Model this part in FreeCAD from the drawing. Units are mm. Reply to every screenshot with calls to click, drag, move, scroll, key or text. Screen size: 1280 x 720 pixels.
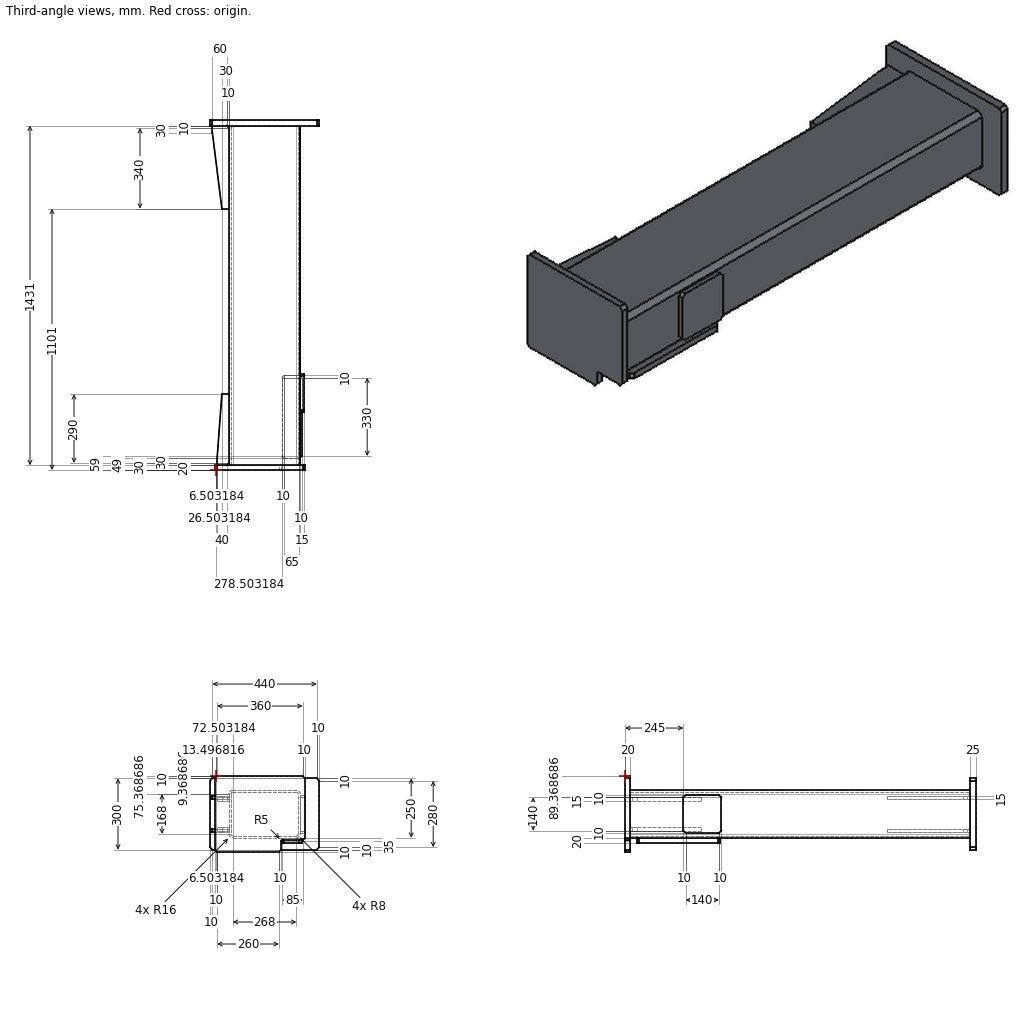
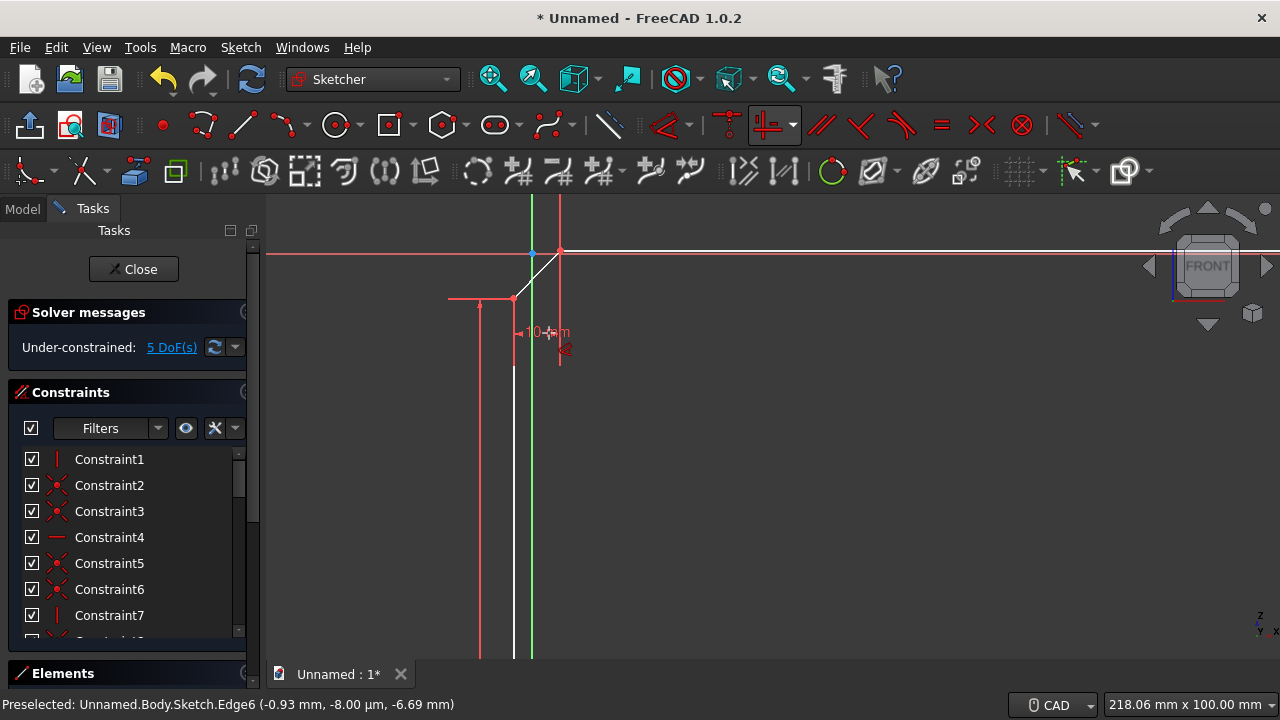
click(546, 265)
click(480, 275)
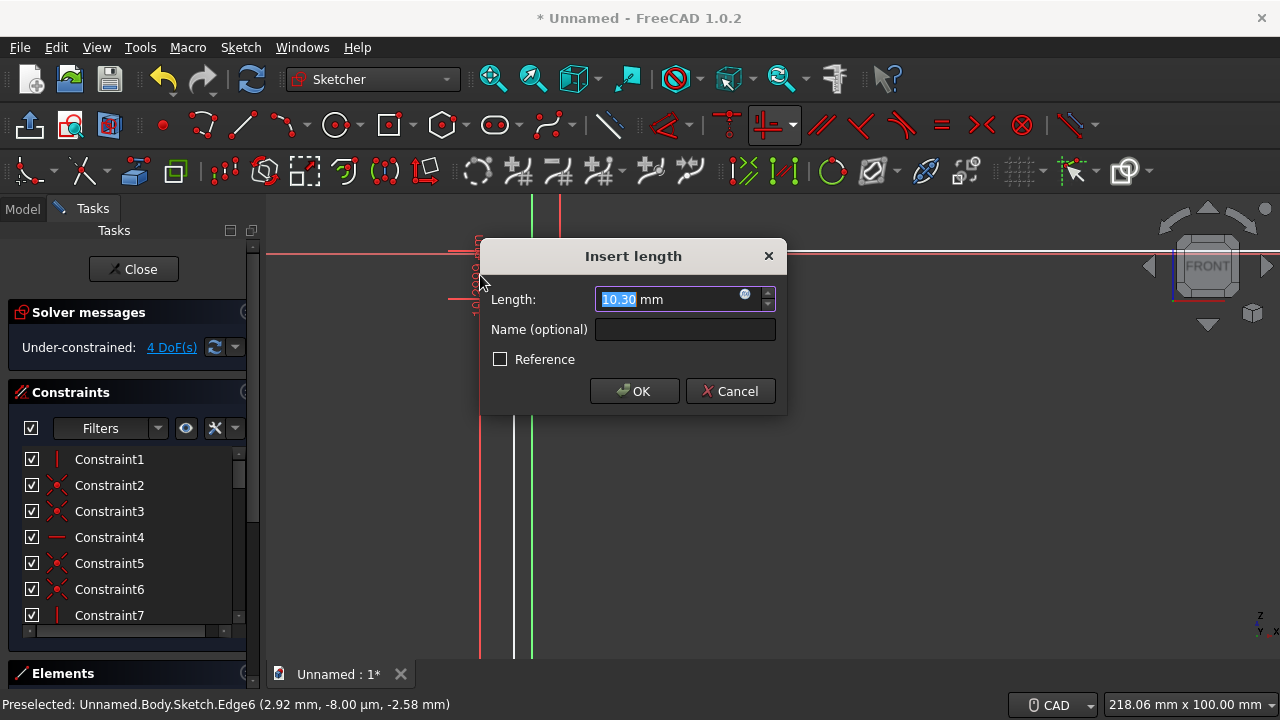
text(10)
key(Return)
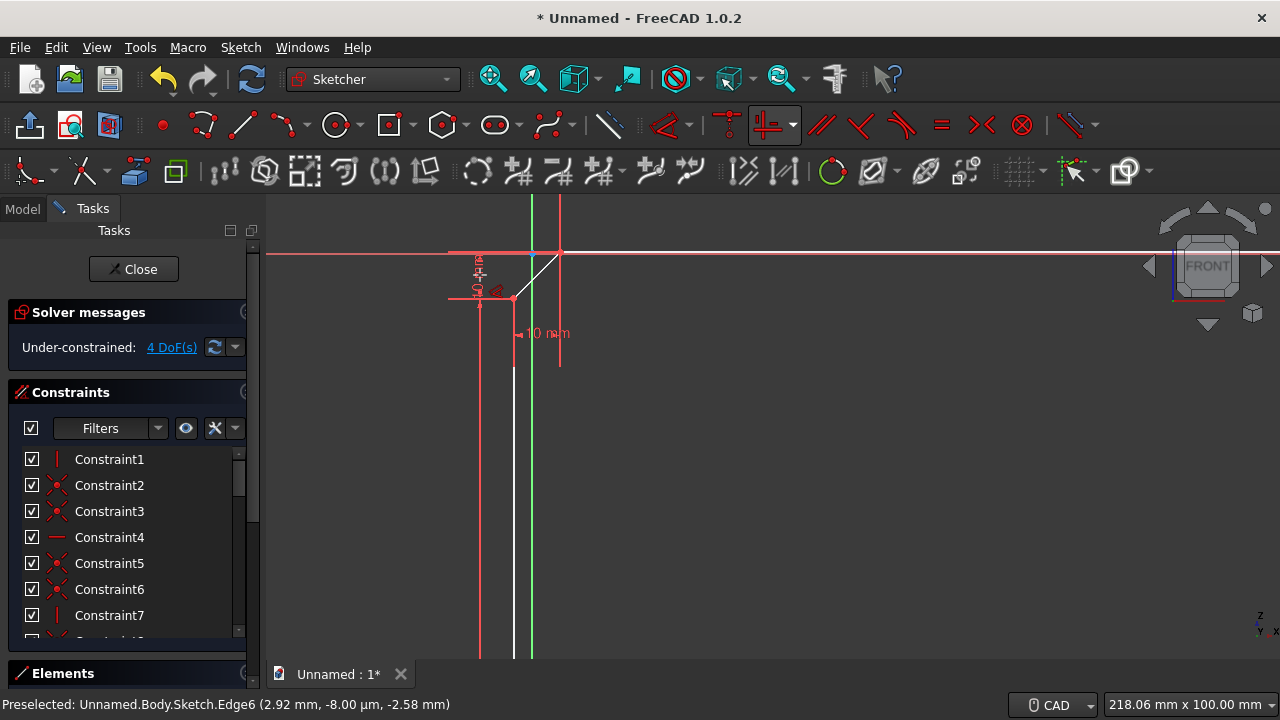
scroll(529, 283, down, 8)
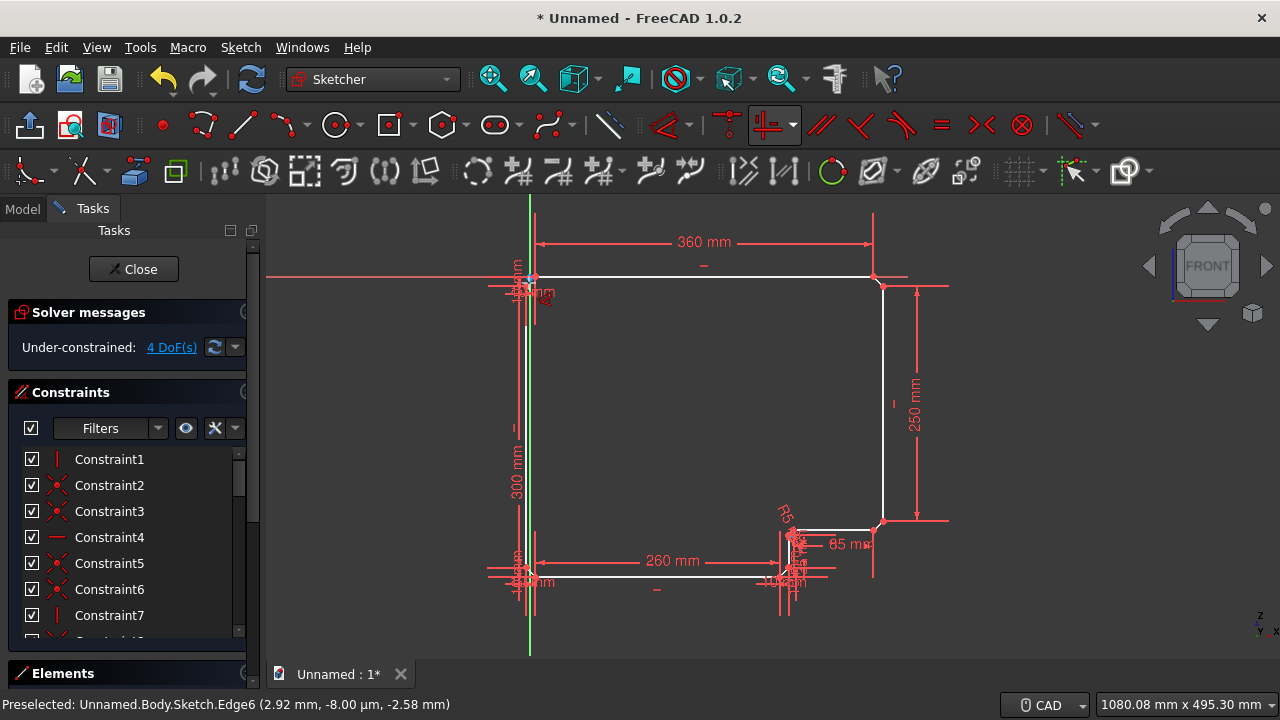
scroll(876, 280, up, 9)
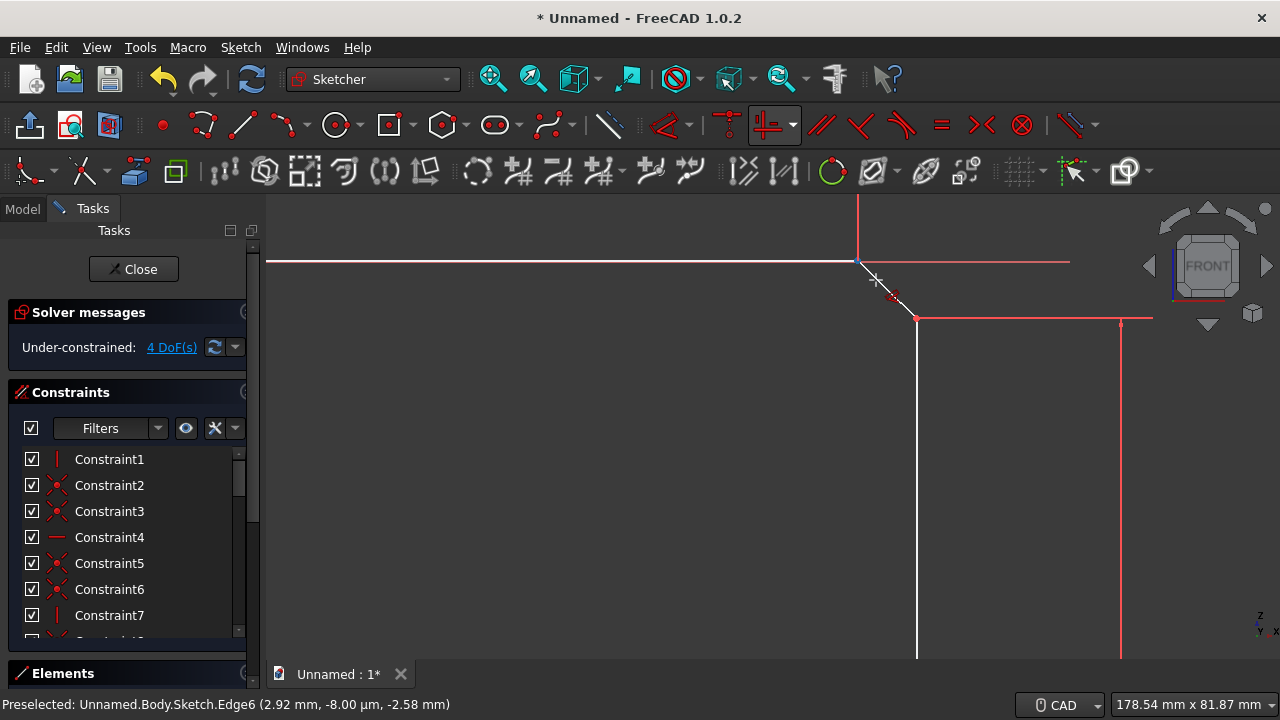
click(875, 278)
click(887, 227)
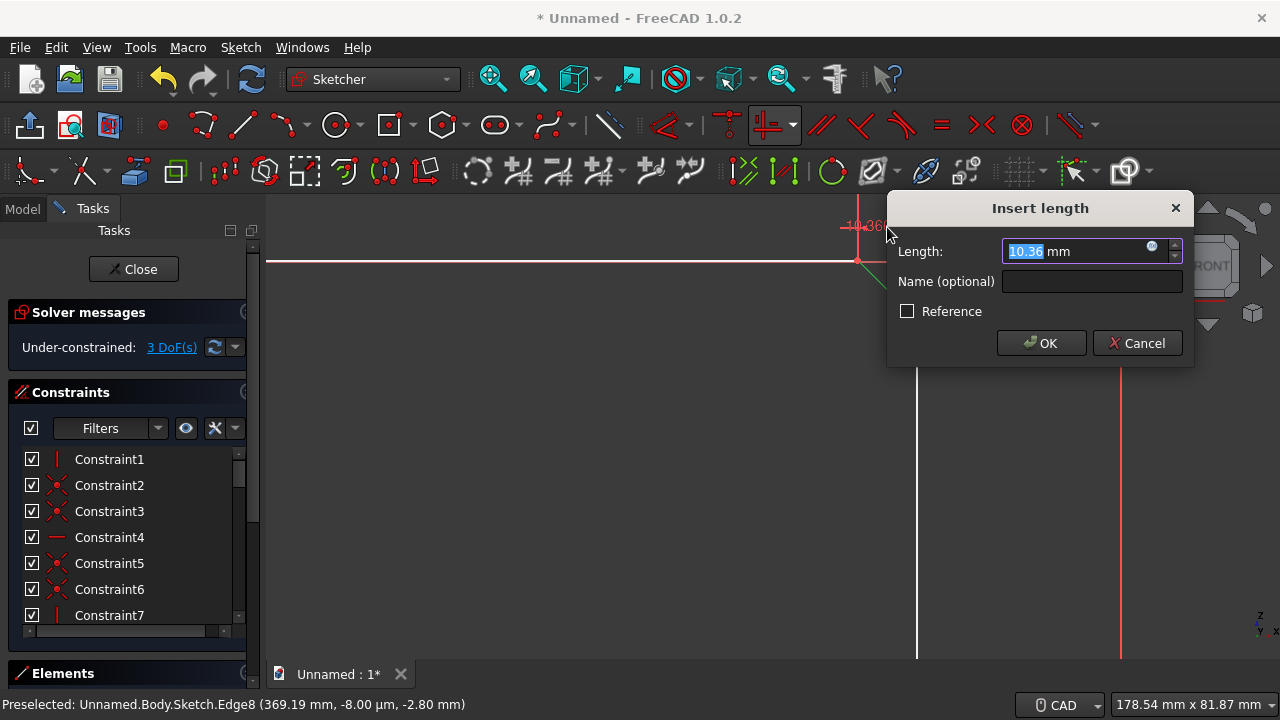
text(10)
key(Return)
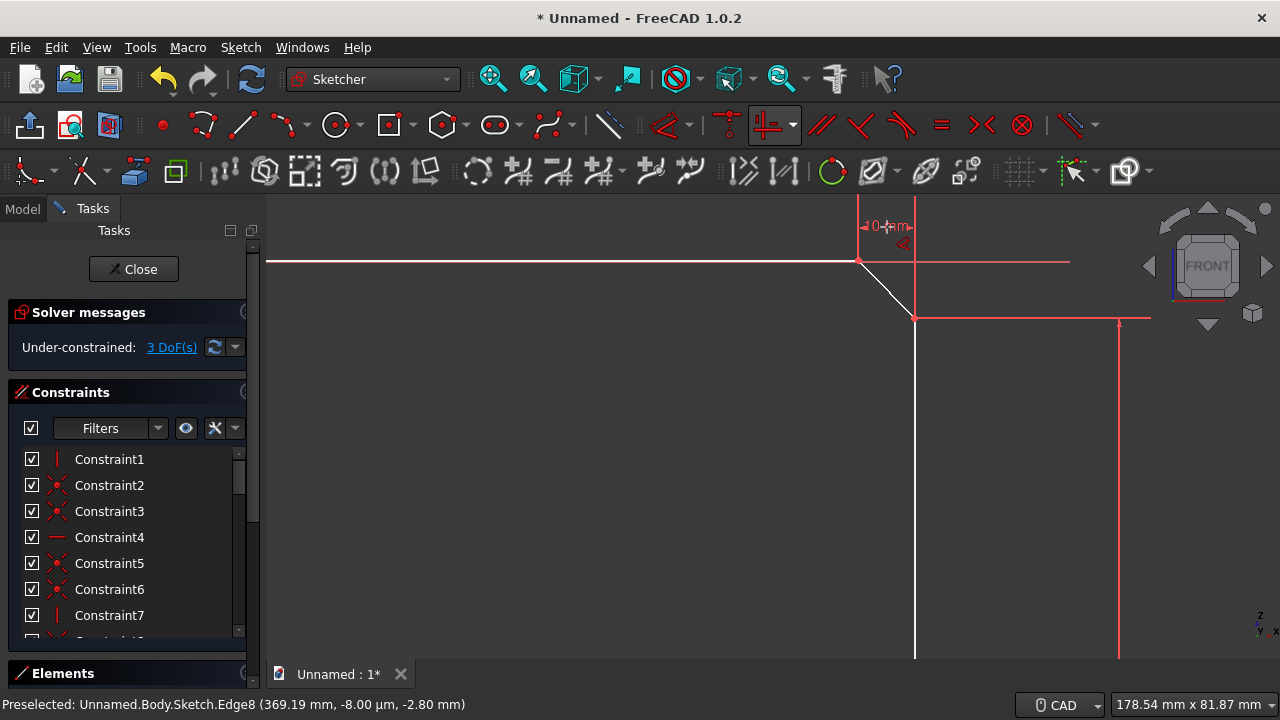
click(875, 278)
click(949, 289)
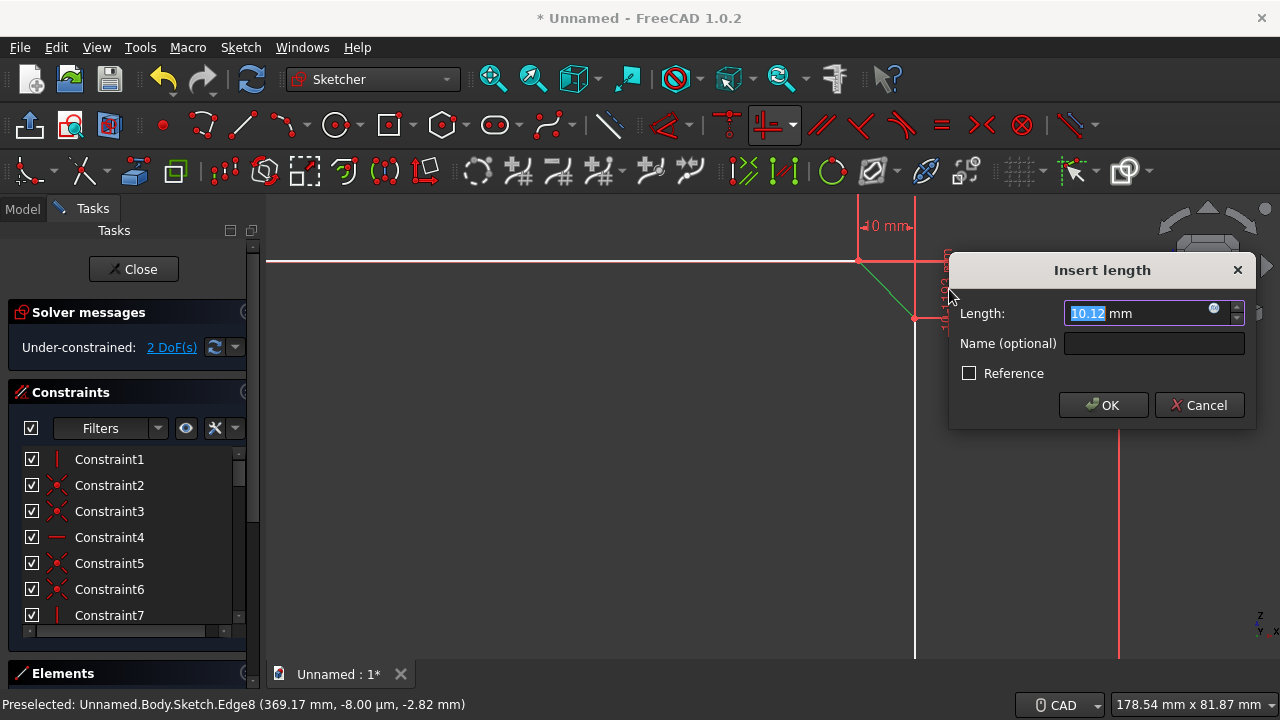
text(10)
key(Return)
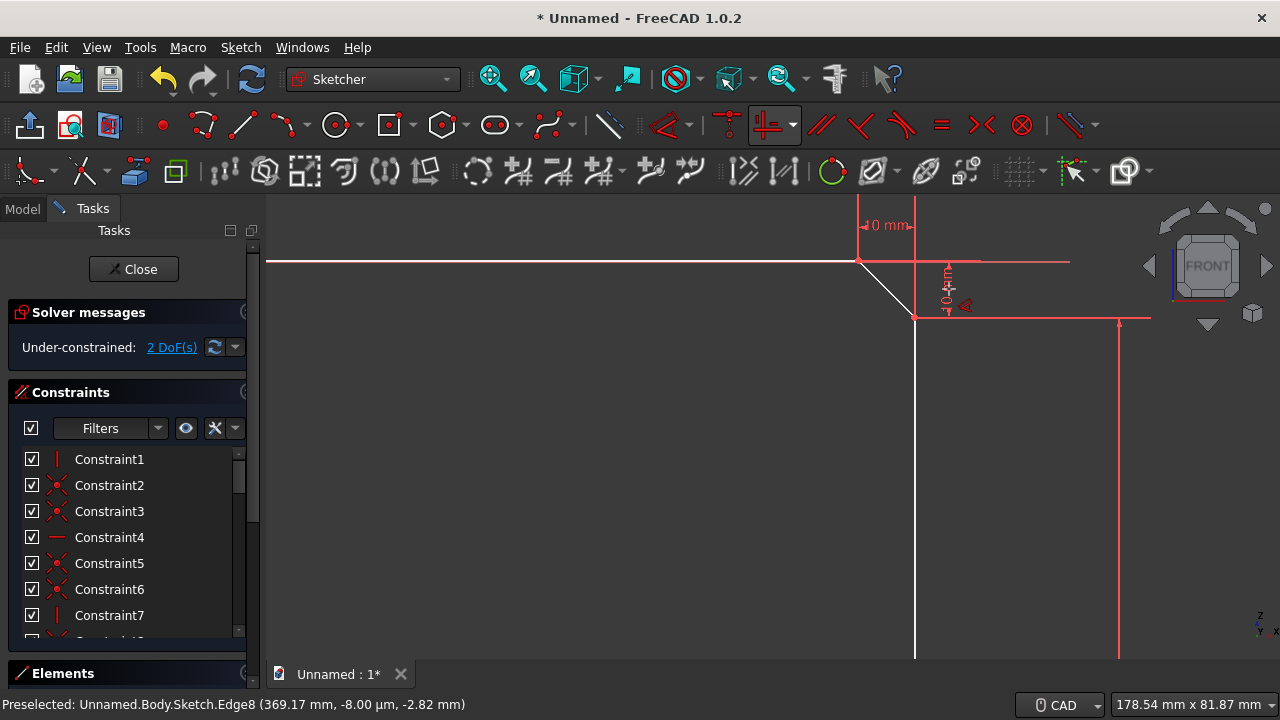
scroll(876, 280, down, 9)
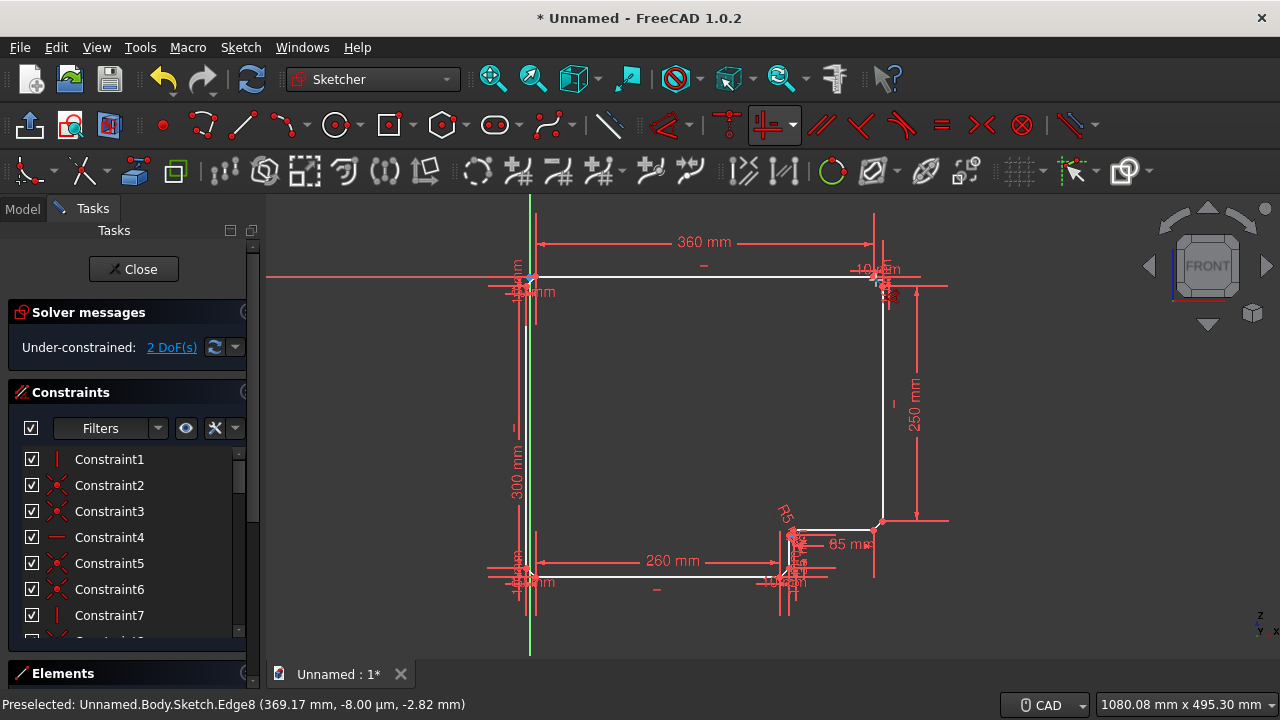
scroll(536, 577, up, 10)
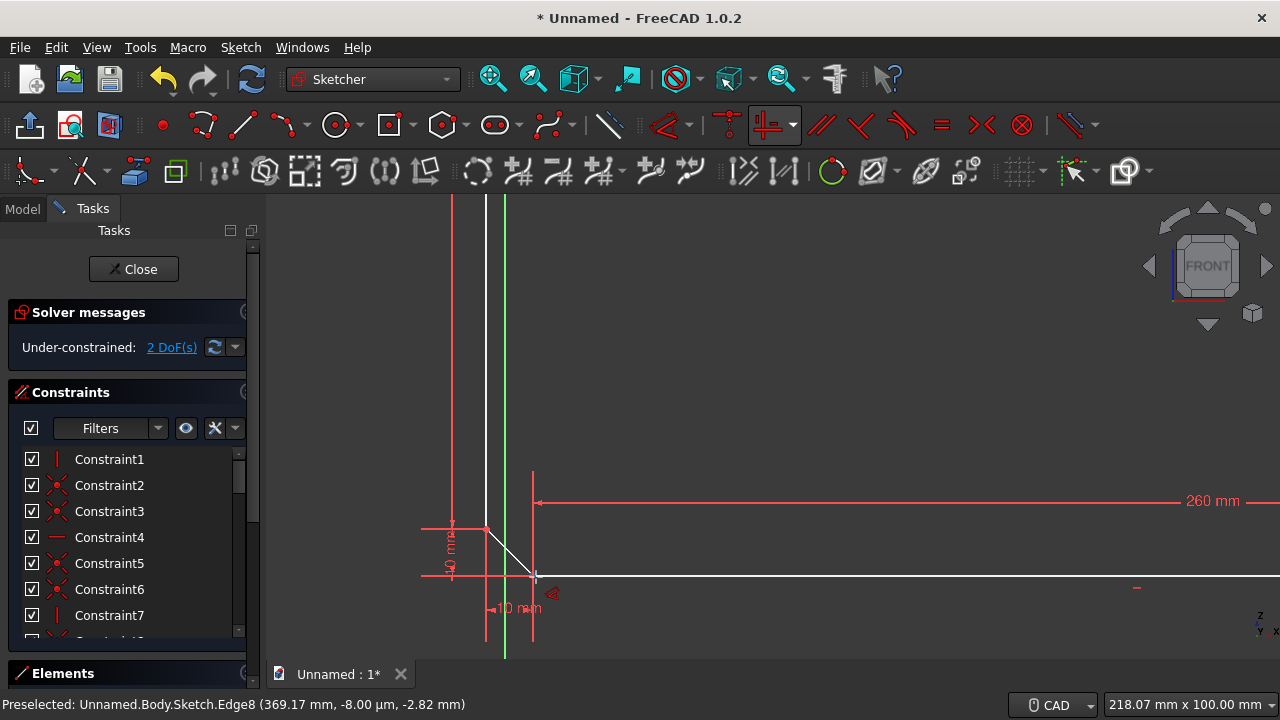
click(531, 575)
click(510, 609)